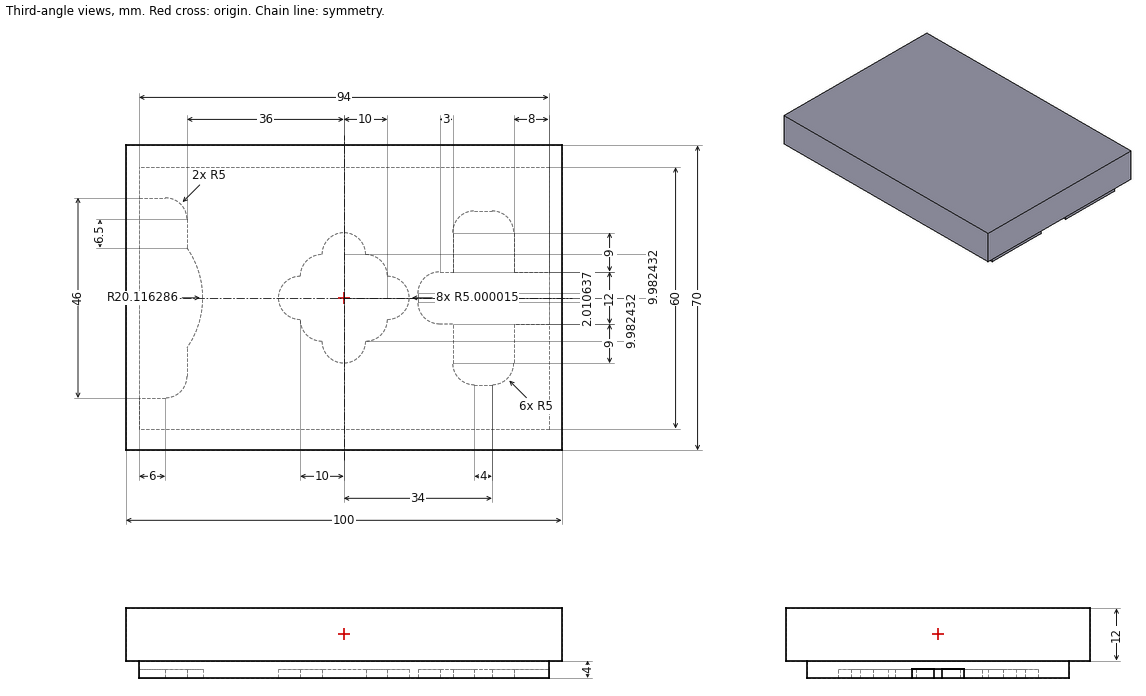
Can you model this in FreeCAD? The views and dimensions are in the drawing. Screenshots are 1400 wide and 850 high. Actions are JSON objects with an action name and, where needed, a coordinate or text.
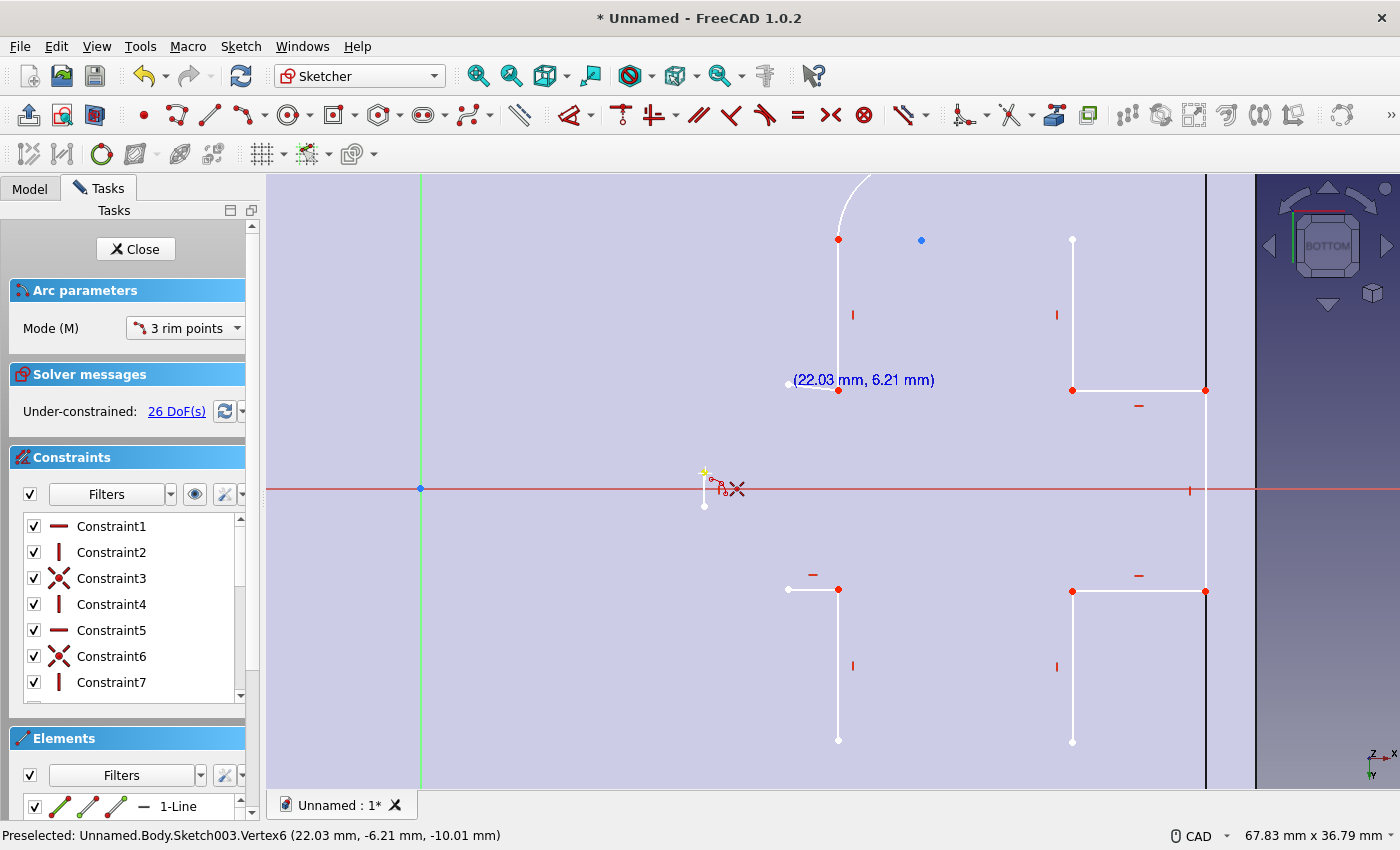
{"action": "left_click", "coordinate": [704, 473]}
{"action": "left_click", "coordinate": [729, 413]}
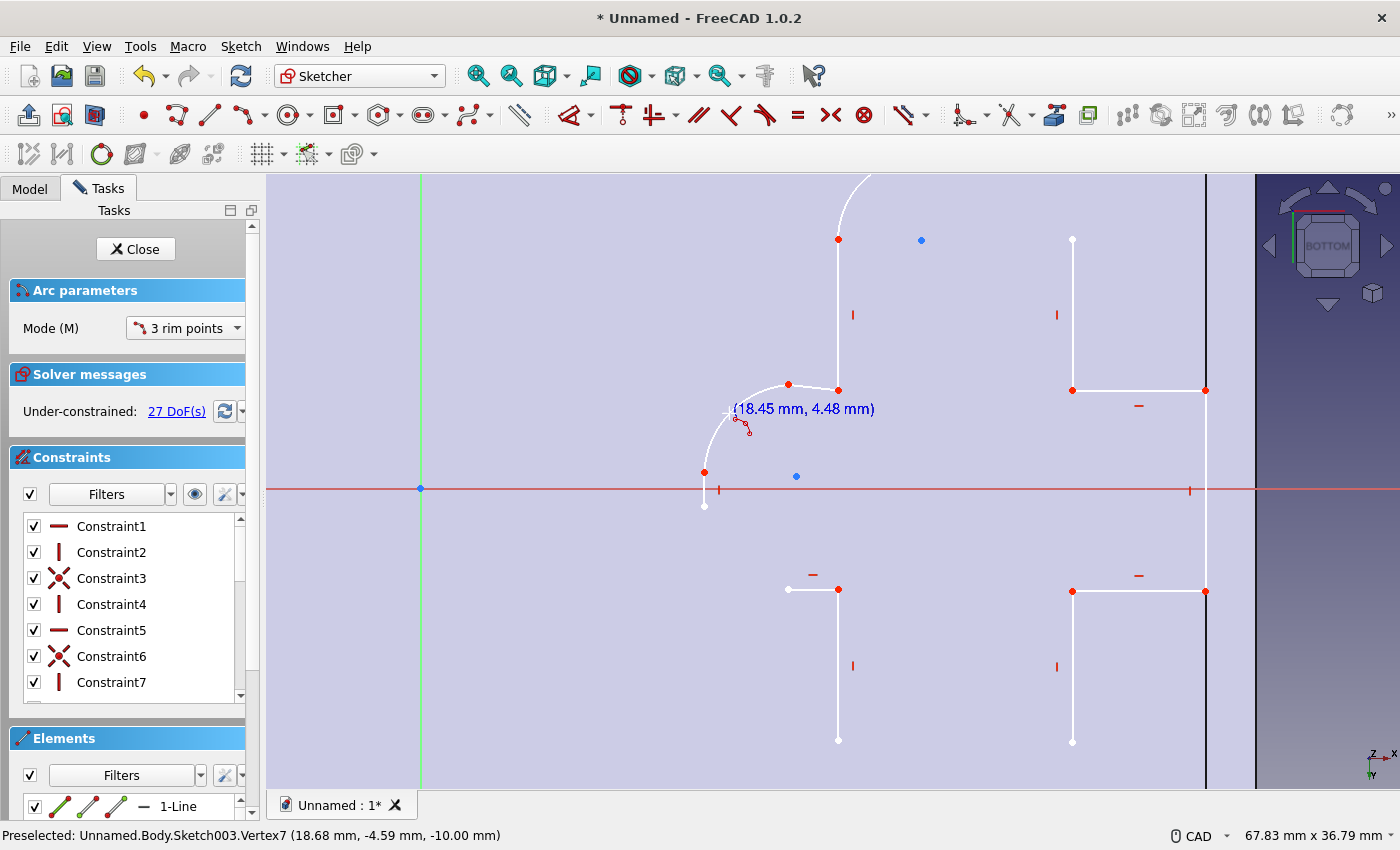
{"action": "left_click", "coordinate": [704, 507]}
{"action": "left_click", "coordinate": [788, 590]}
{"action": "left_click", "coordinate": [729, 565]}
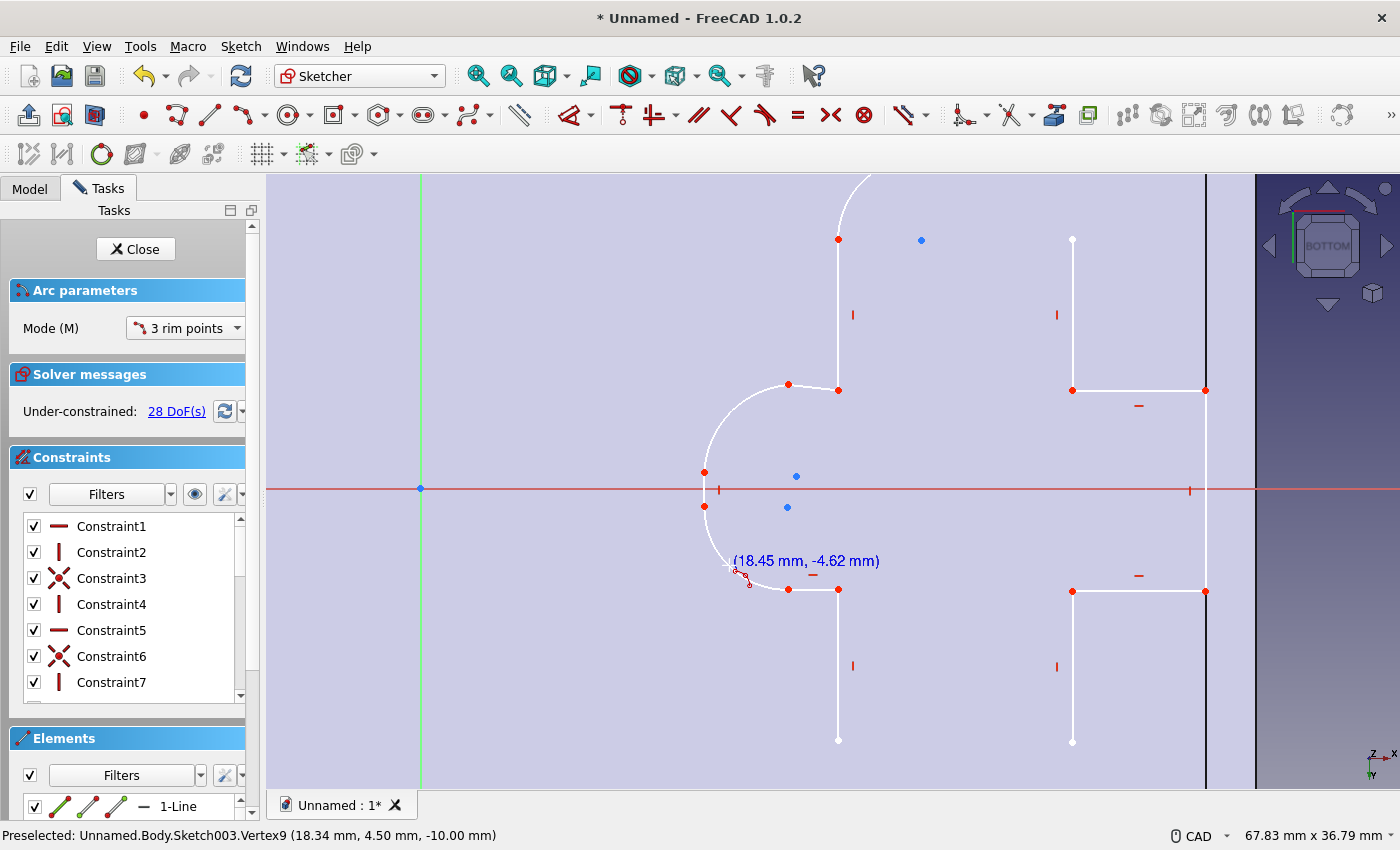
{"action": "left_click", "coordinate": [838, 741]}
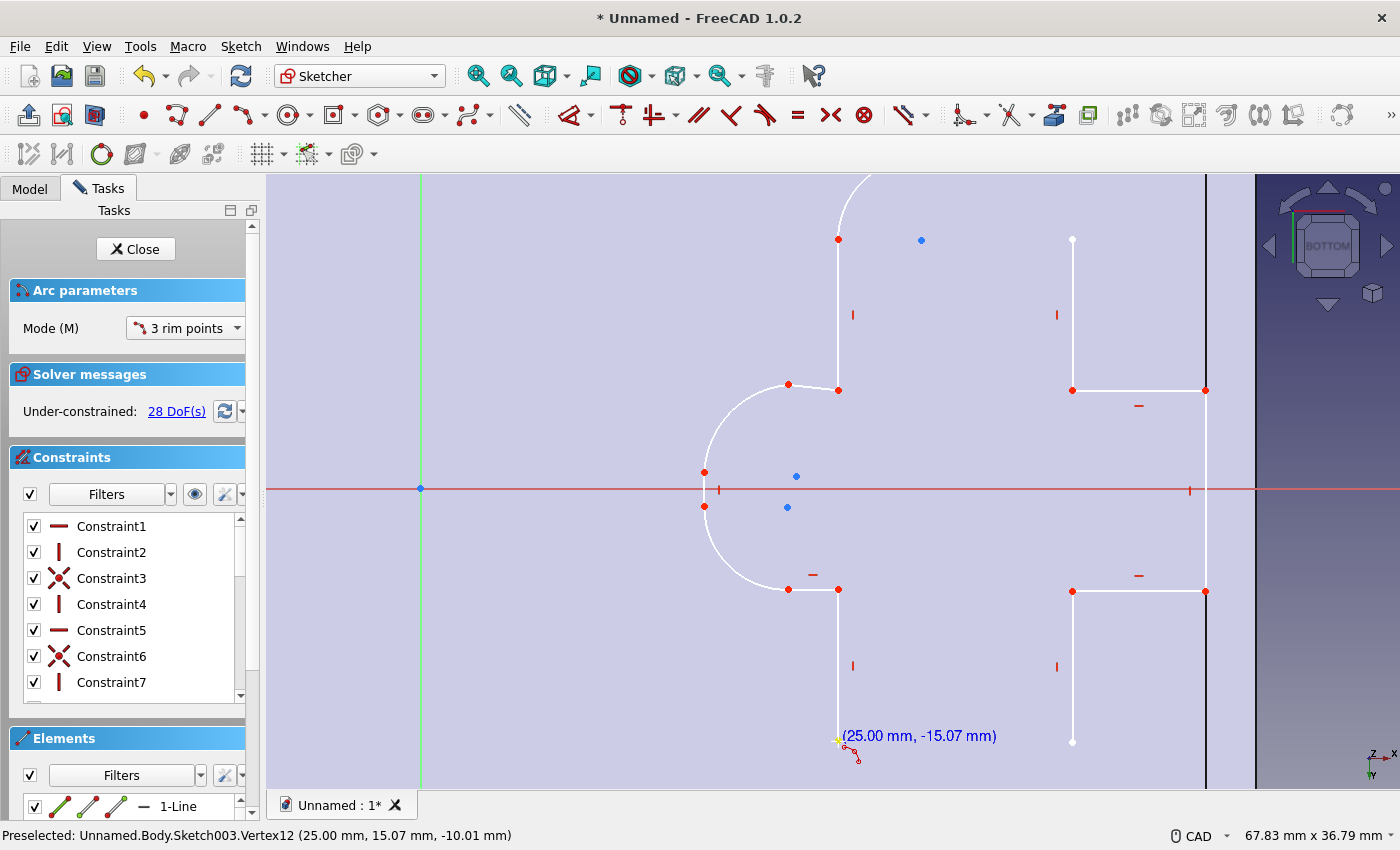
{"action": "scroll", "coordinate": [705, 473], "scroll_direction": "down", "scroll_amount": 3}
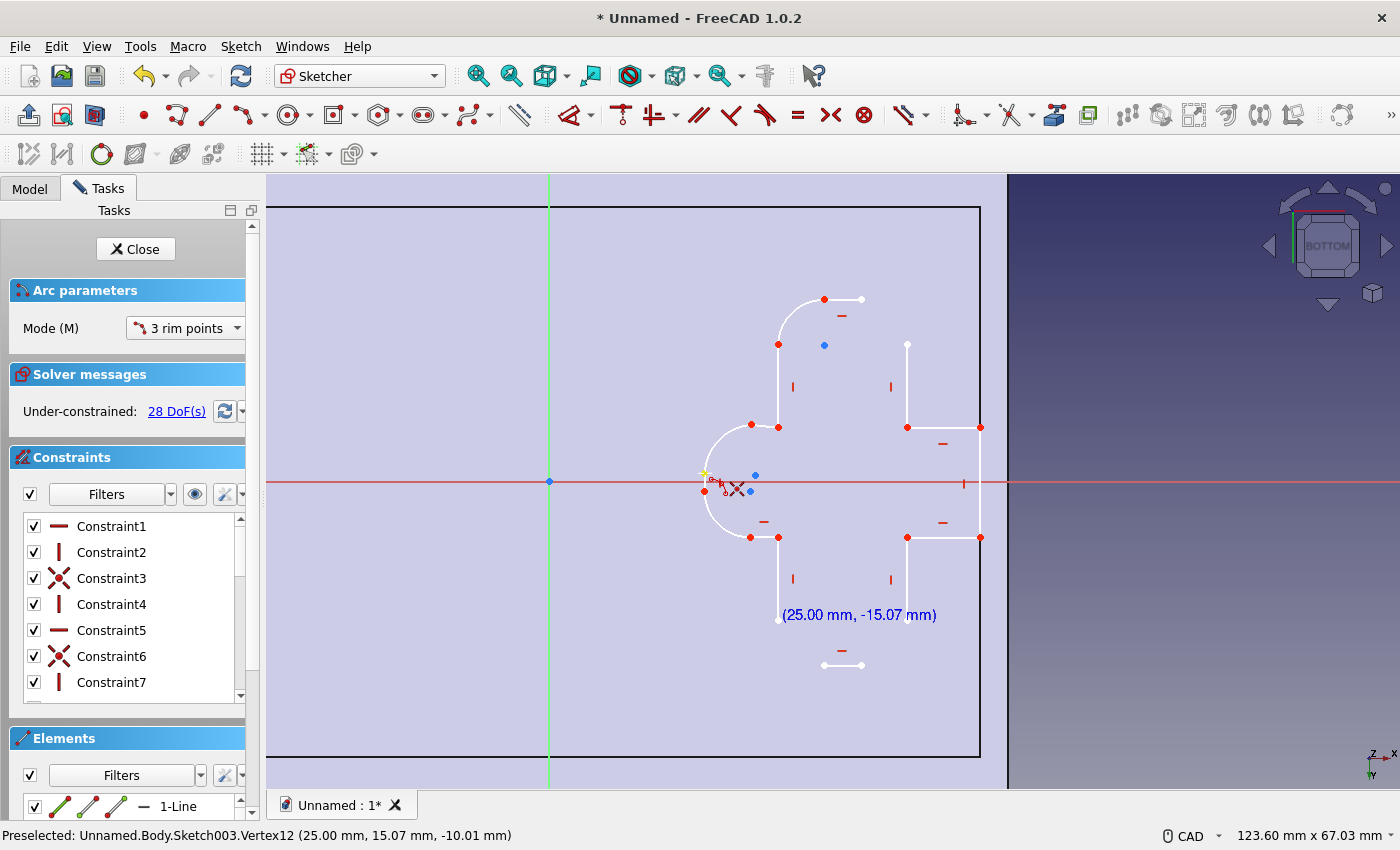
{"action": "left_click", "coordinate": [824, 666]}
{"action": "left_click", "coordinate": [792, 652]}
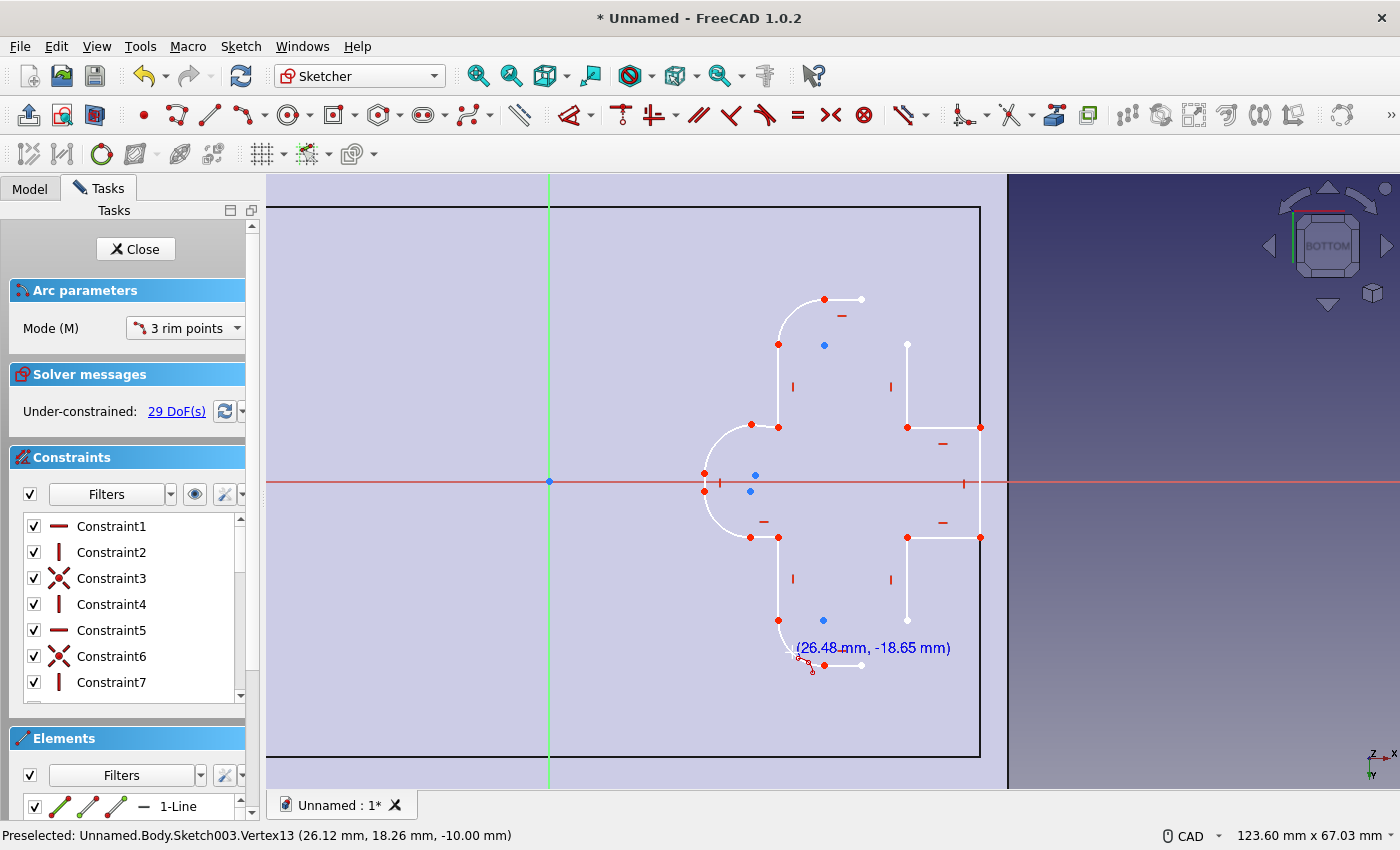
{"action": "left_click", "coordinate": [861, 666]}
{"action": "left_click", "coordinate": [907, 621]}
{"action": "left_click", "coordinate": [893, 652]}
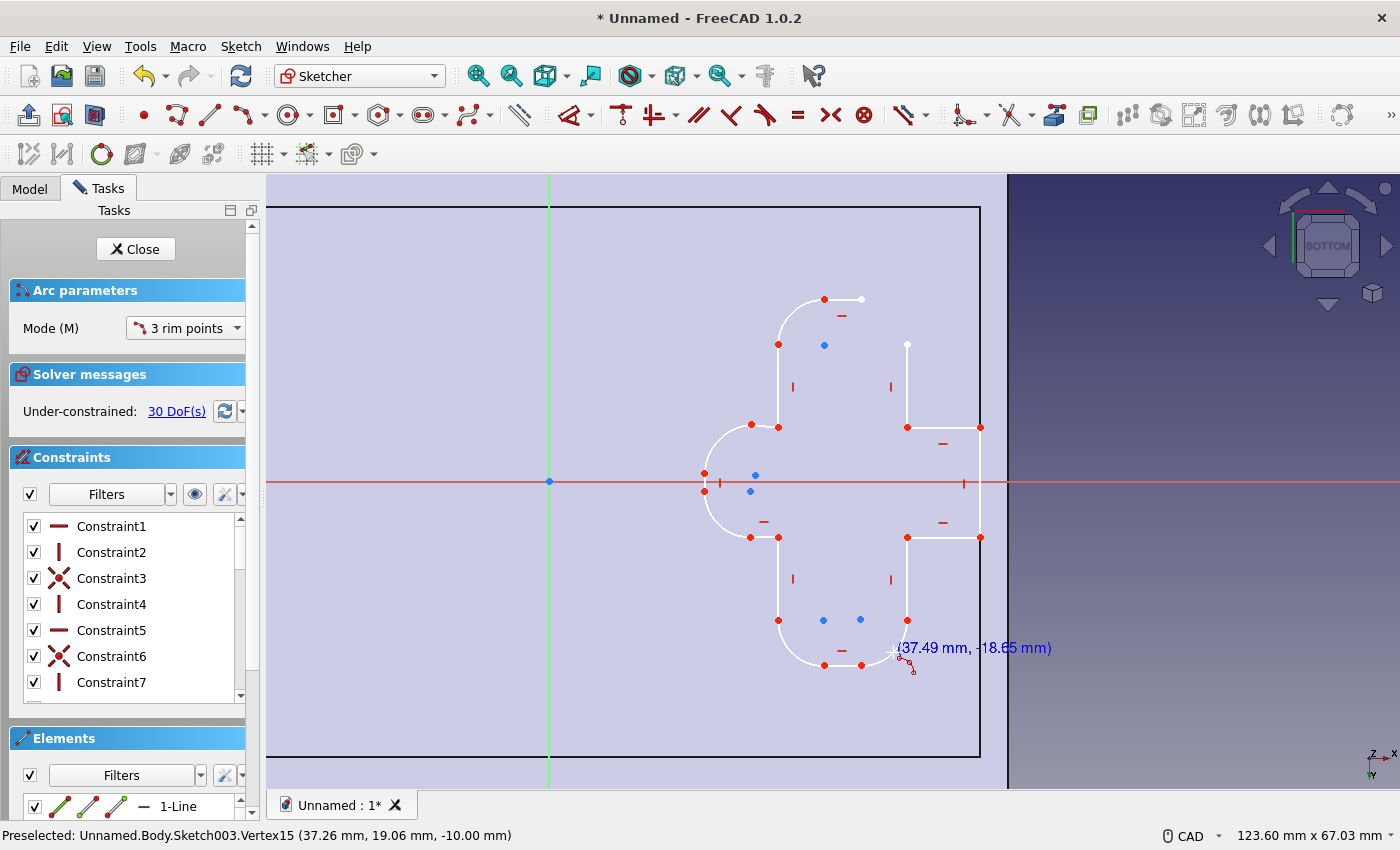
{"action": "left_click", "coordinate": [907, 345]}
{"action": "left_click", "coordinate": [861, 300]}
{"action": "left_click", "coordinate": [893, 312]}
{"action": "key", "text": "Escape"}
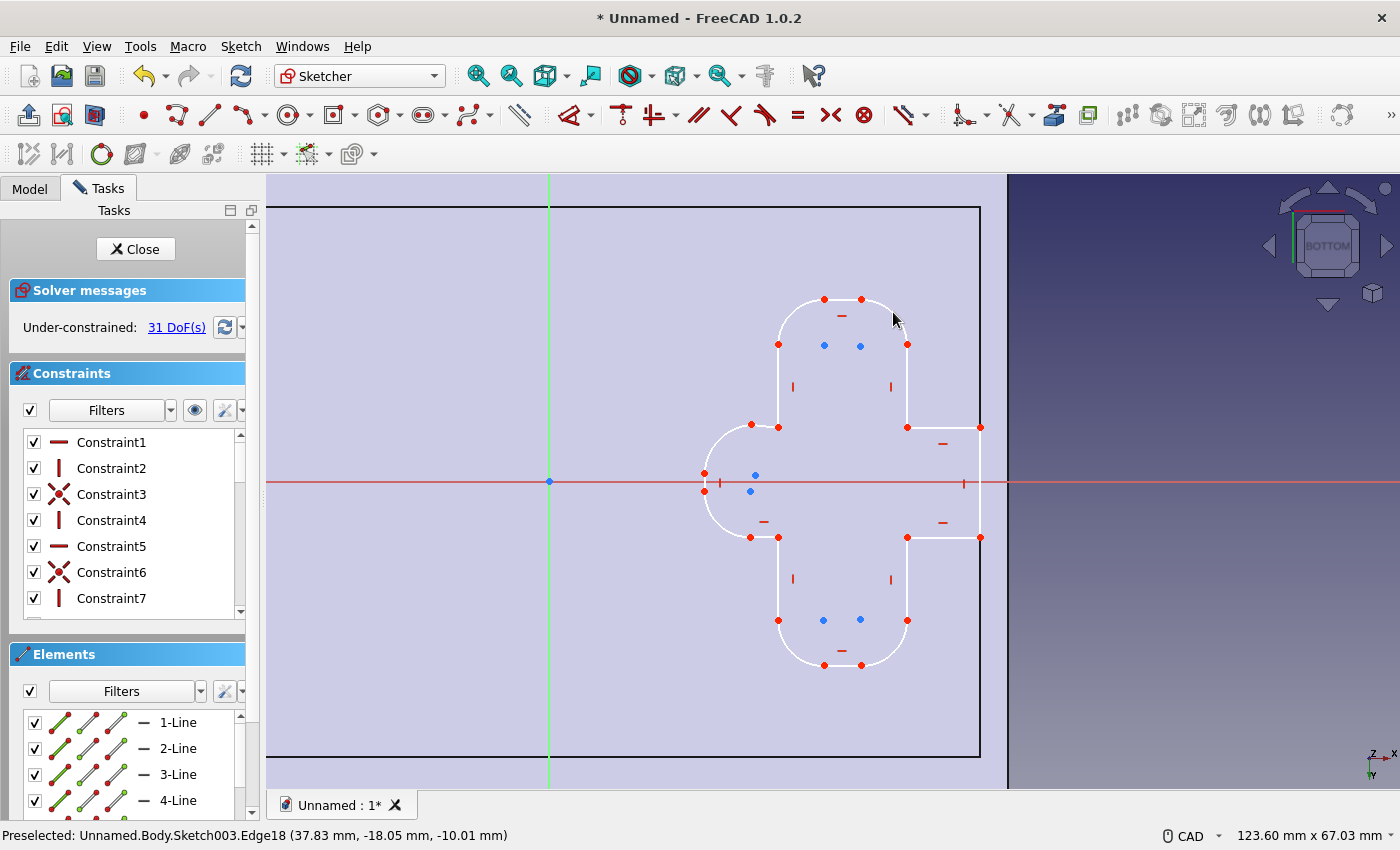
{"action": "scroll", "coordinate": [850, 300], "scroll_direction": "up", "scroll_amount": 2}